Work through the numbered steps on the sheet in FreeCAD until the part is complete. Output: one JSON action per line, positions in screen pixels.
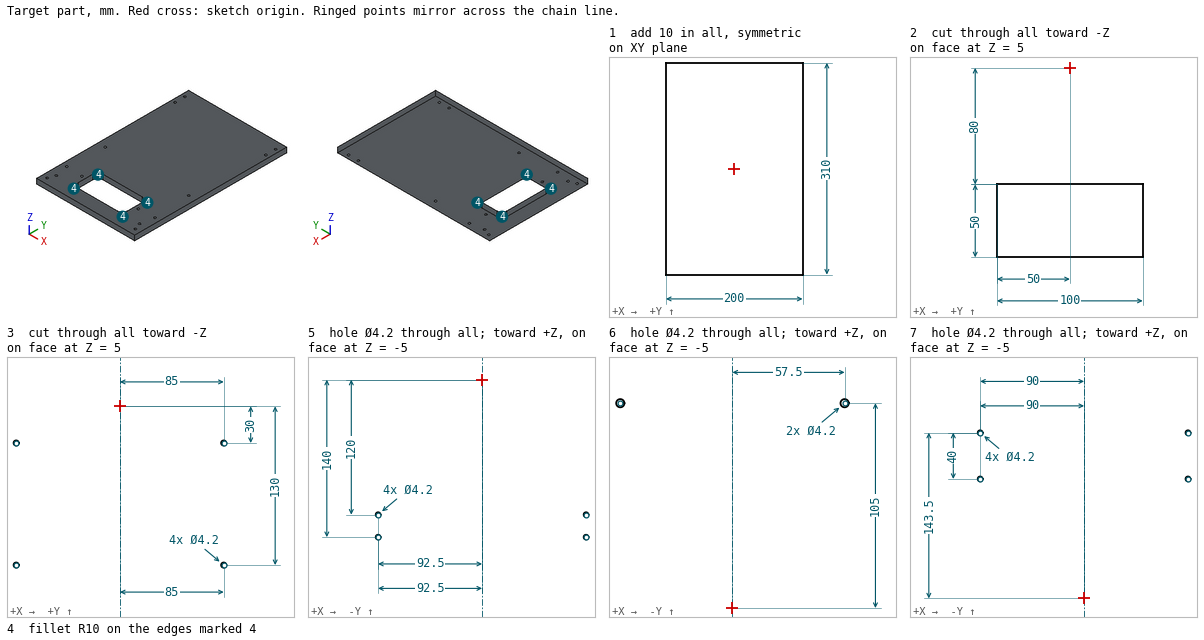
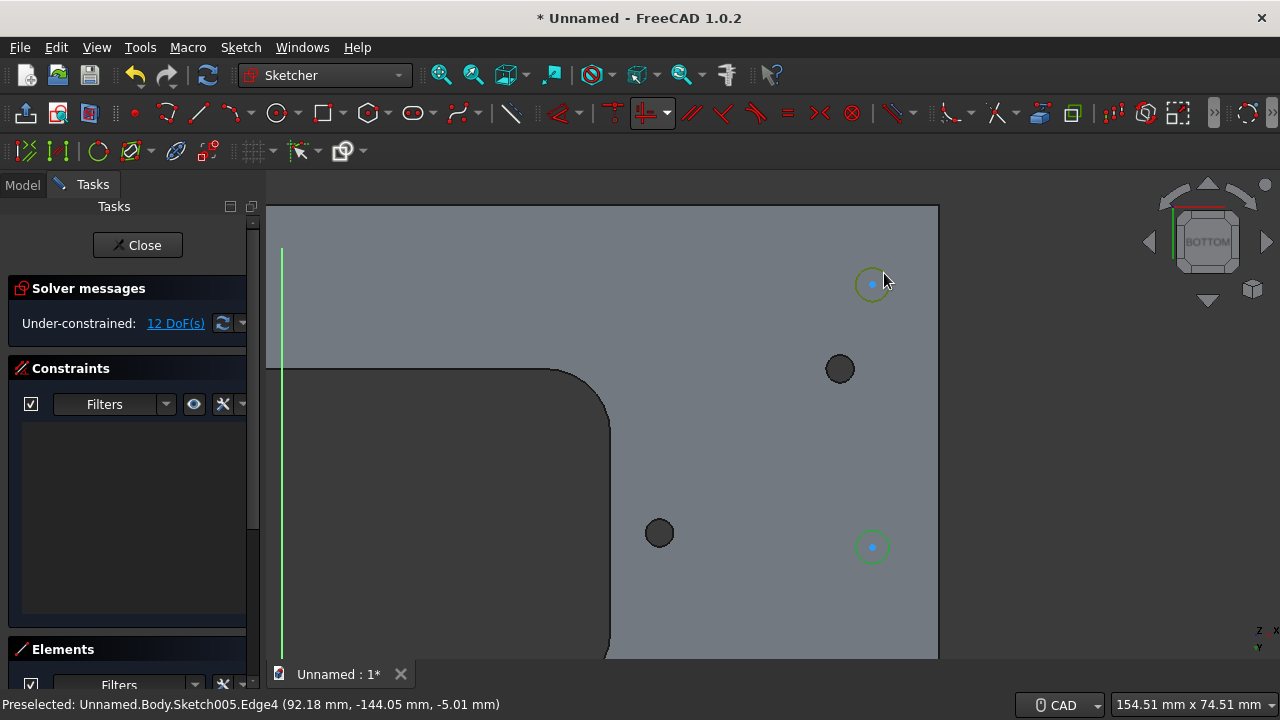
{"action": "left_click", "coordinate": [788, 114]}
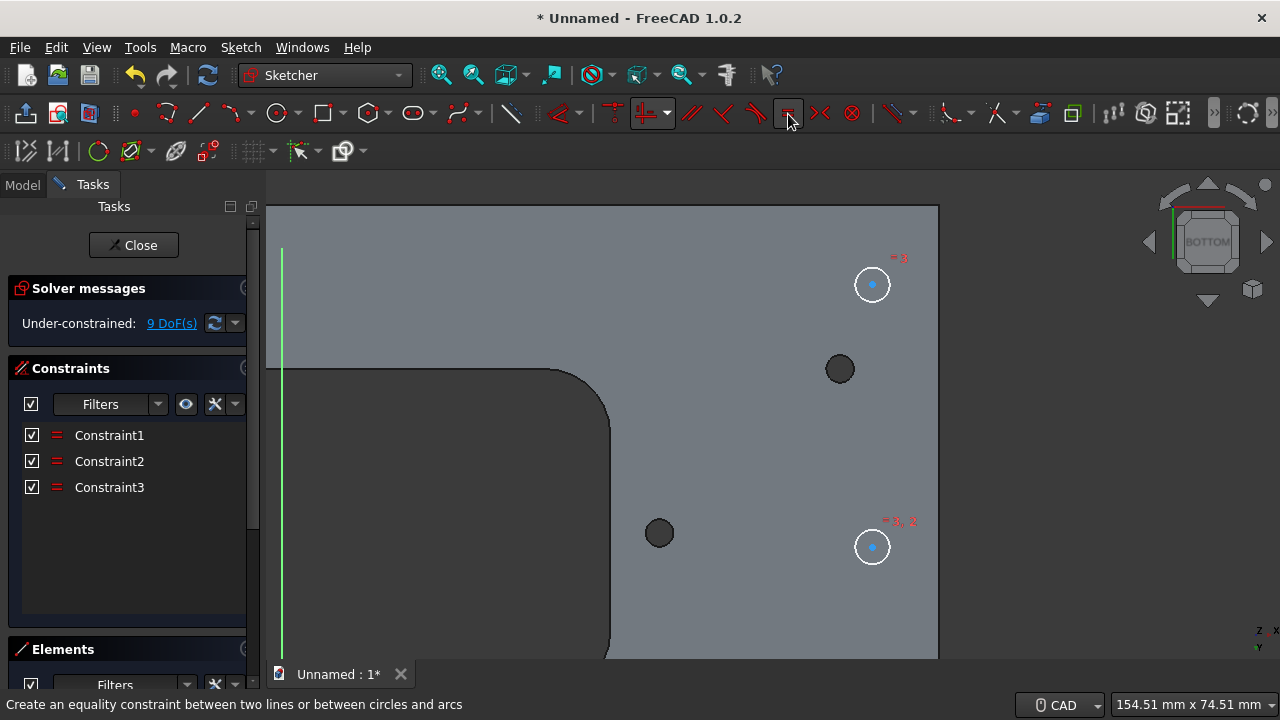
{"action": "scroll", "coordinate": [886, 272], "scroll_direction": "down", "scroll_amount": 6}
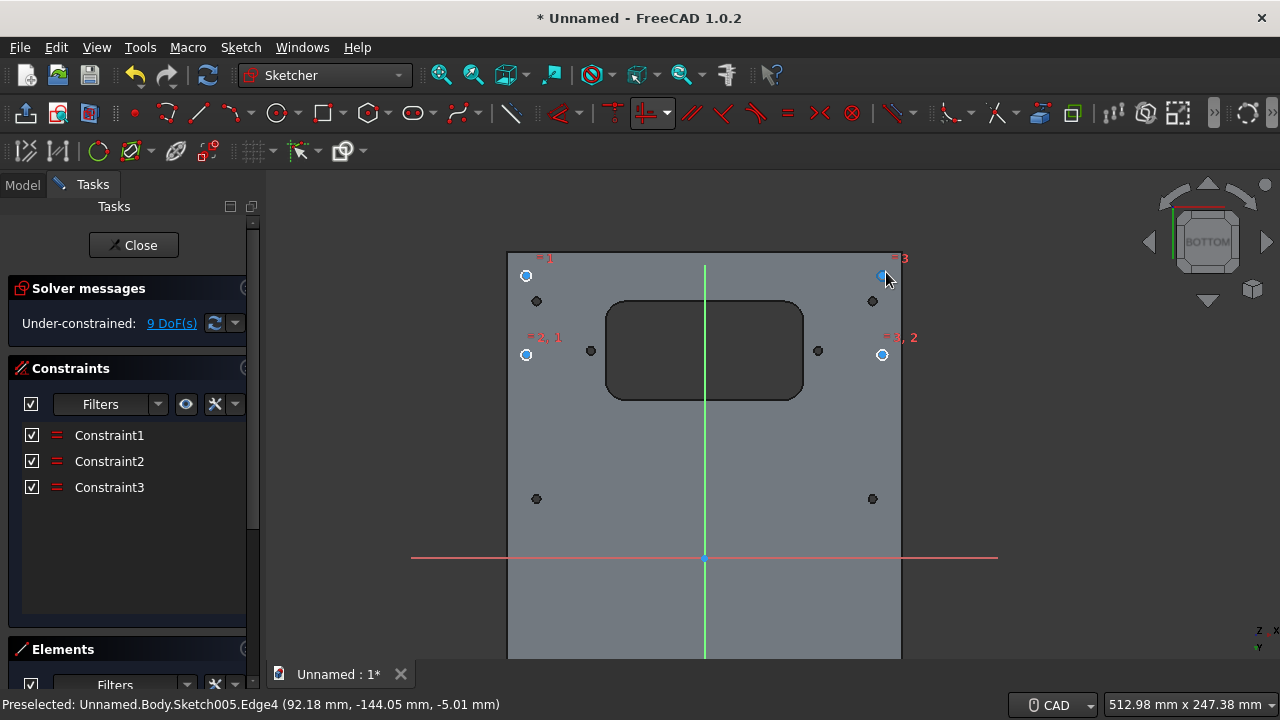
{"action": "left_click", "coordinate": [526, 355]}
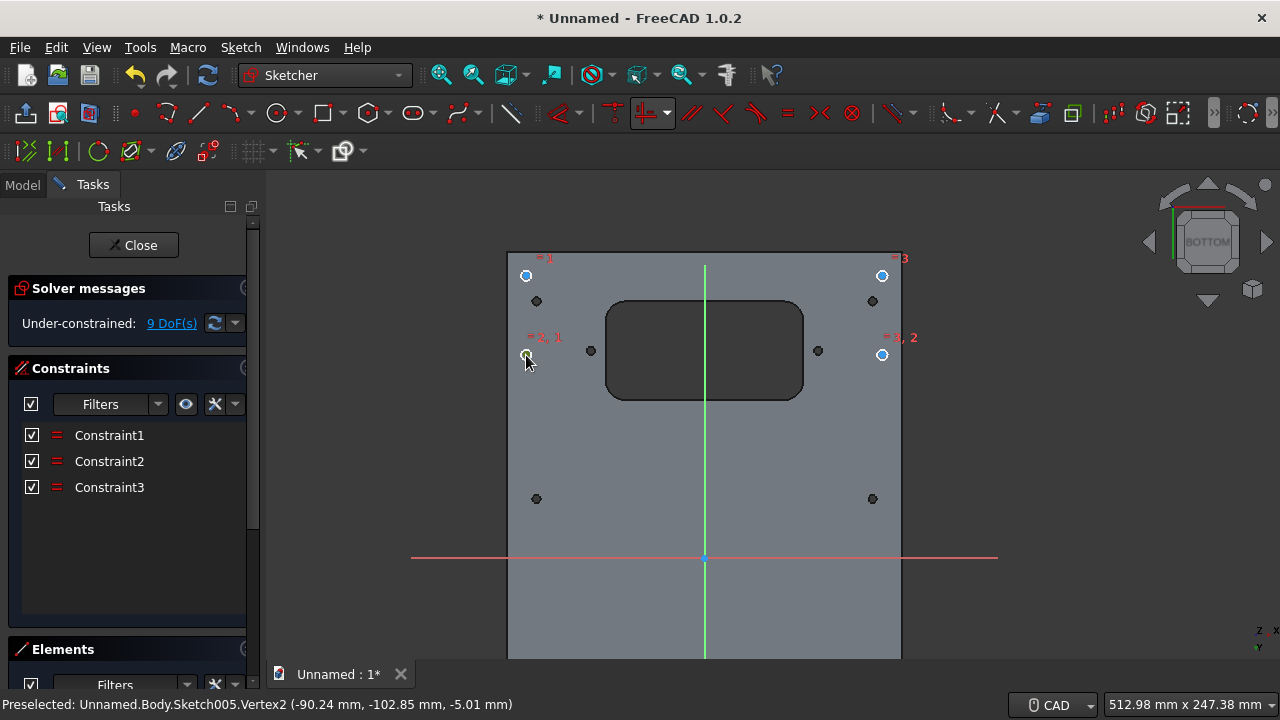
{"action": "left_click", "coordinate": [882, 355]}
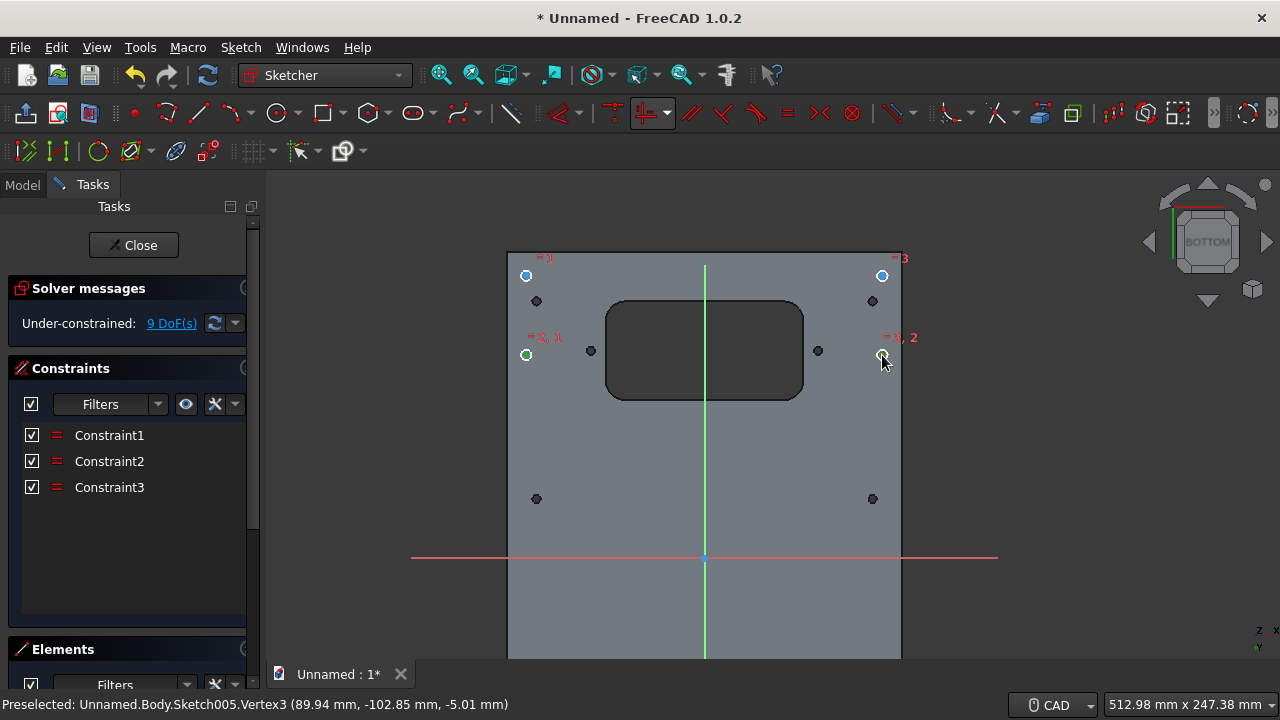
{"action": "left_click", "coordinate": [705, 600]}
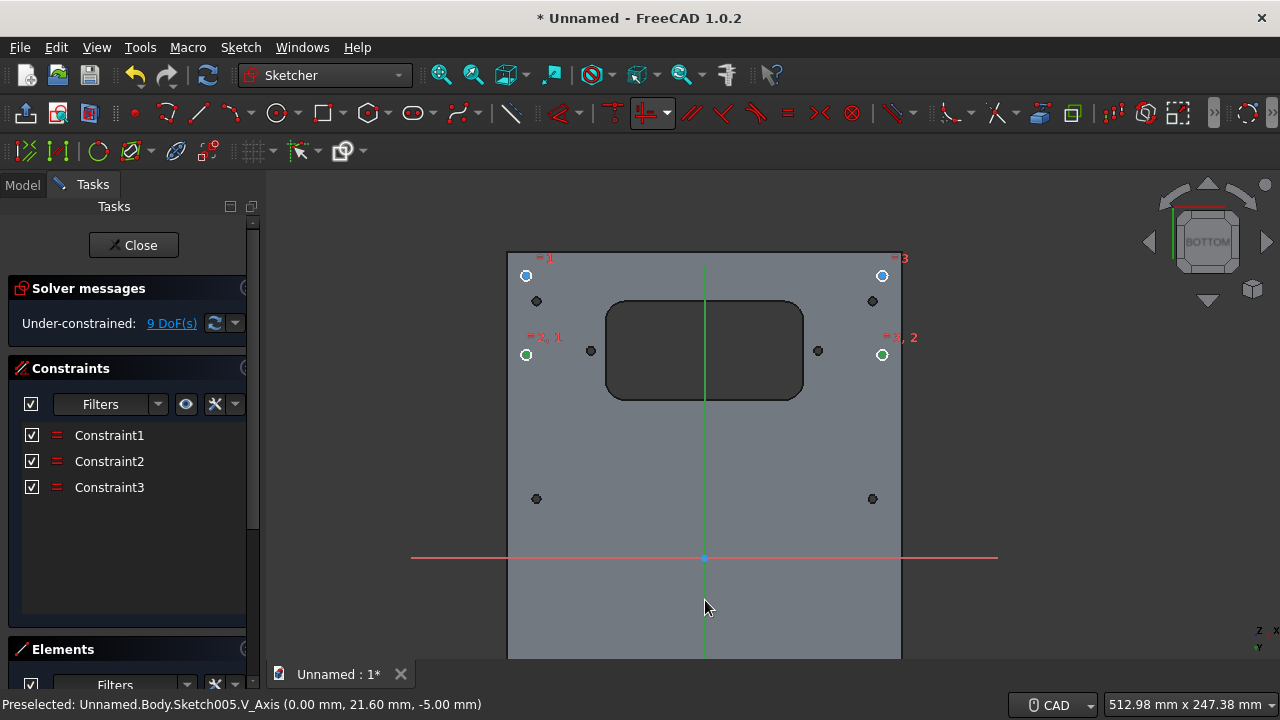
{"action": "left_click", "coordinate": [820, 114]}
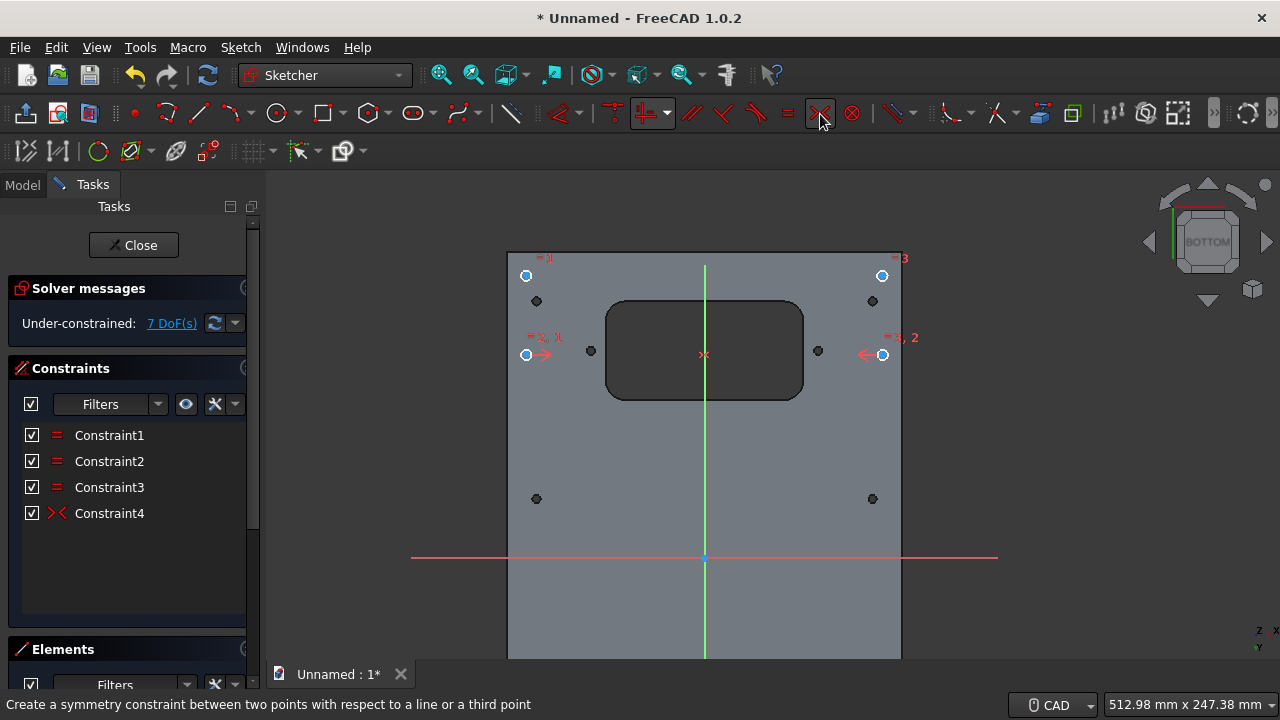
{"action": "left_click", "coordinate": [526, 276]}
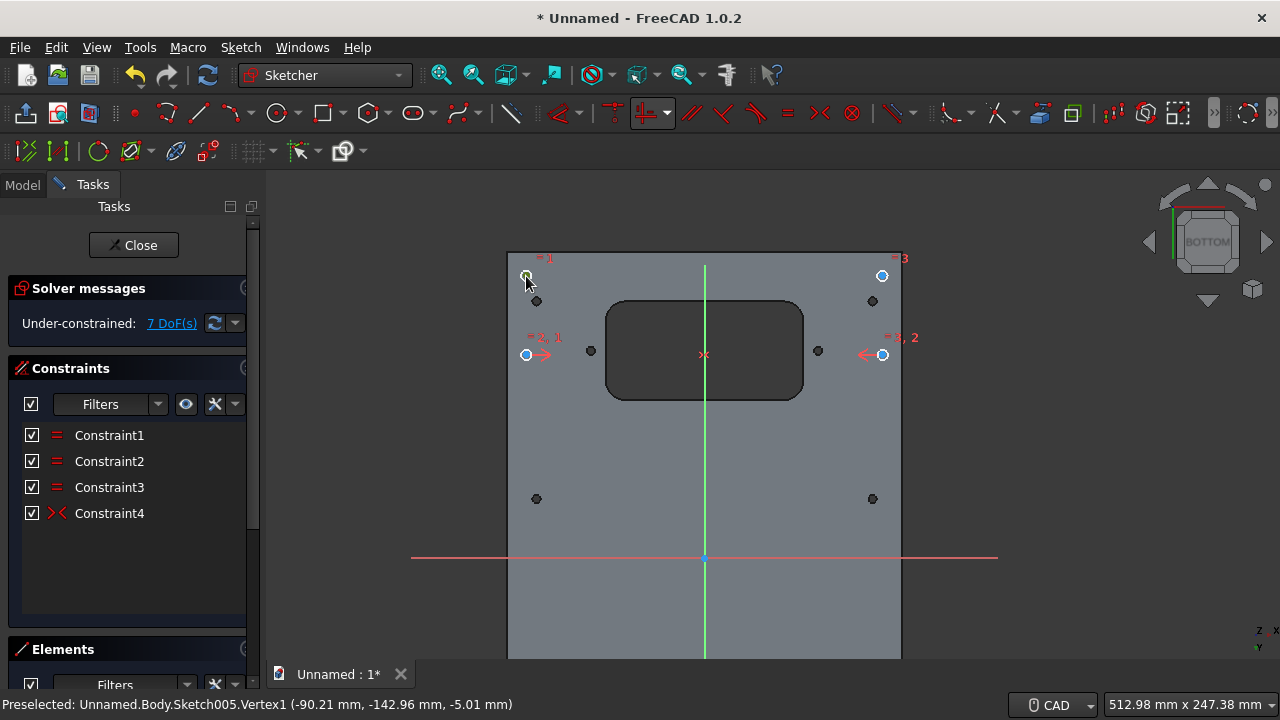
{"action": "left_click", "coordinate": [882, 276]}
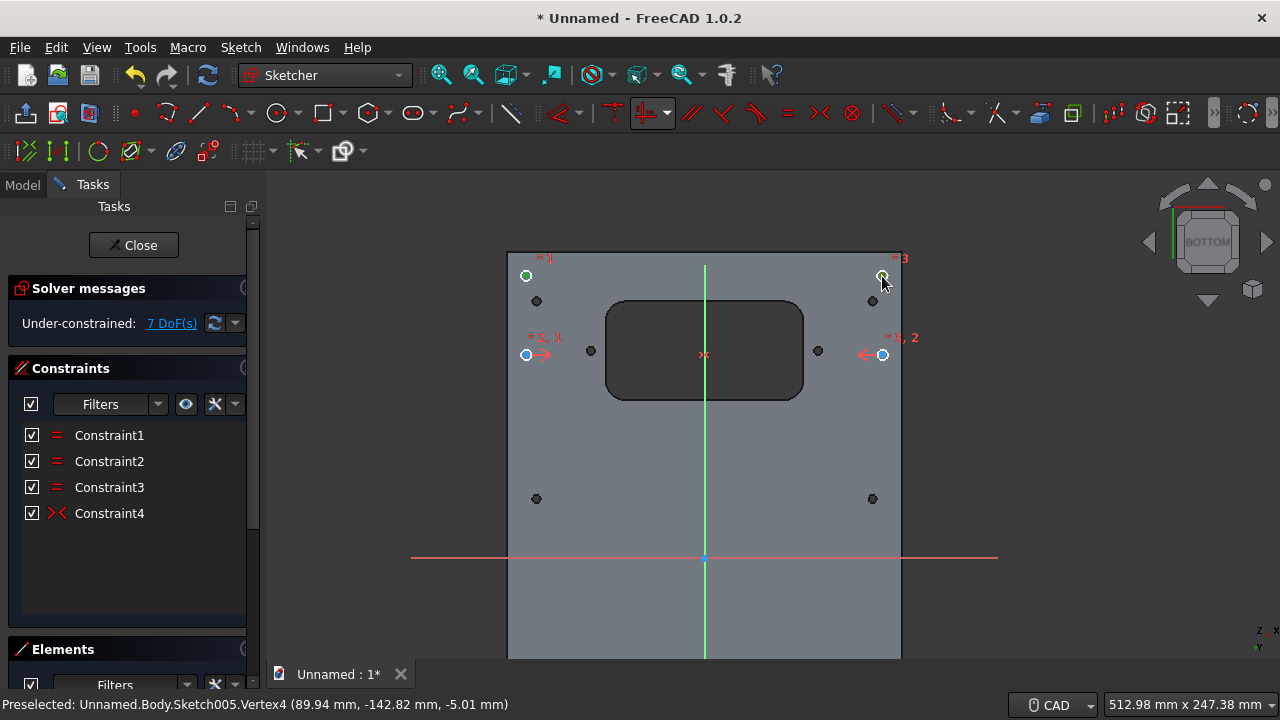
{"action": "left_click", "coordinate": [705, 600]}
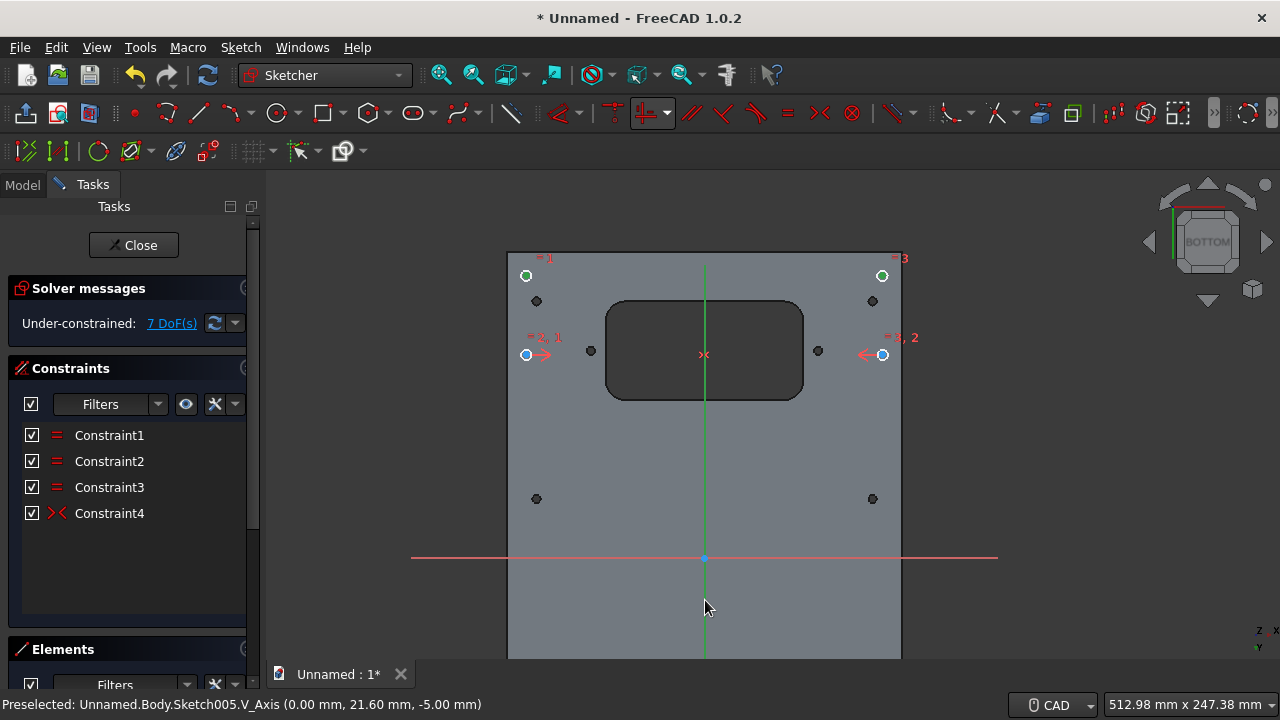
{"action": "key", "text": "s"}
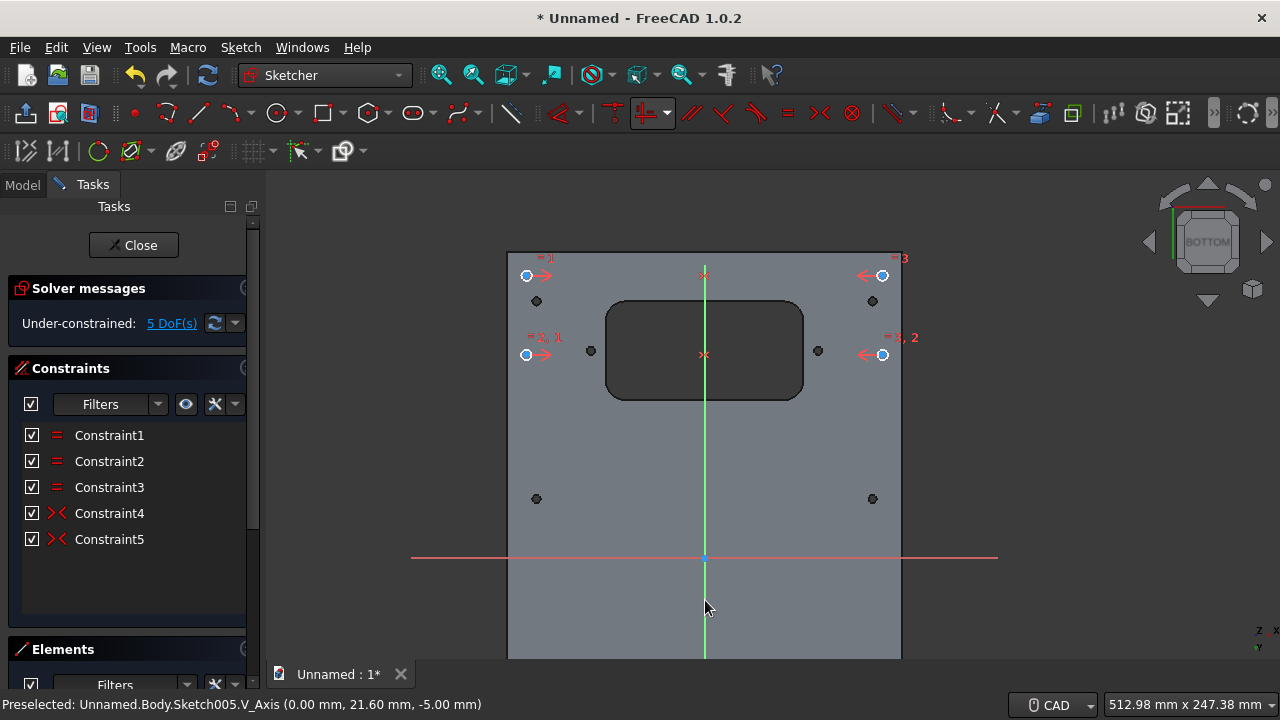
{"action": "left_click", "coordinate": [558, 114]}